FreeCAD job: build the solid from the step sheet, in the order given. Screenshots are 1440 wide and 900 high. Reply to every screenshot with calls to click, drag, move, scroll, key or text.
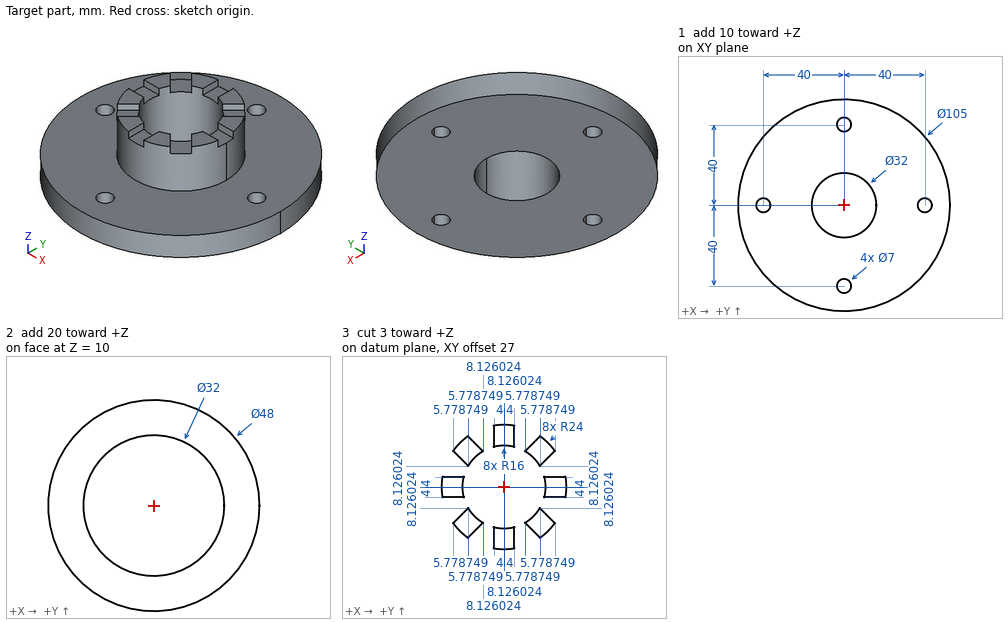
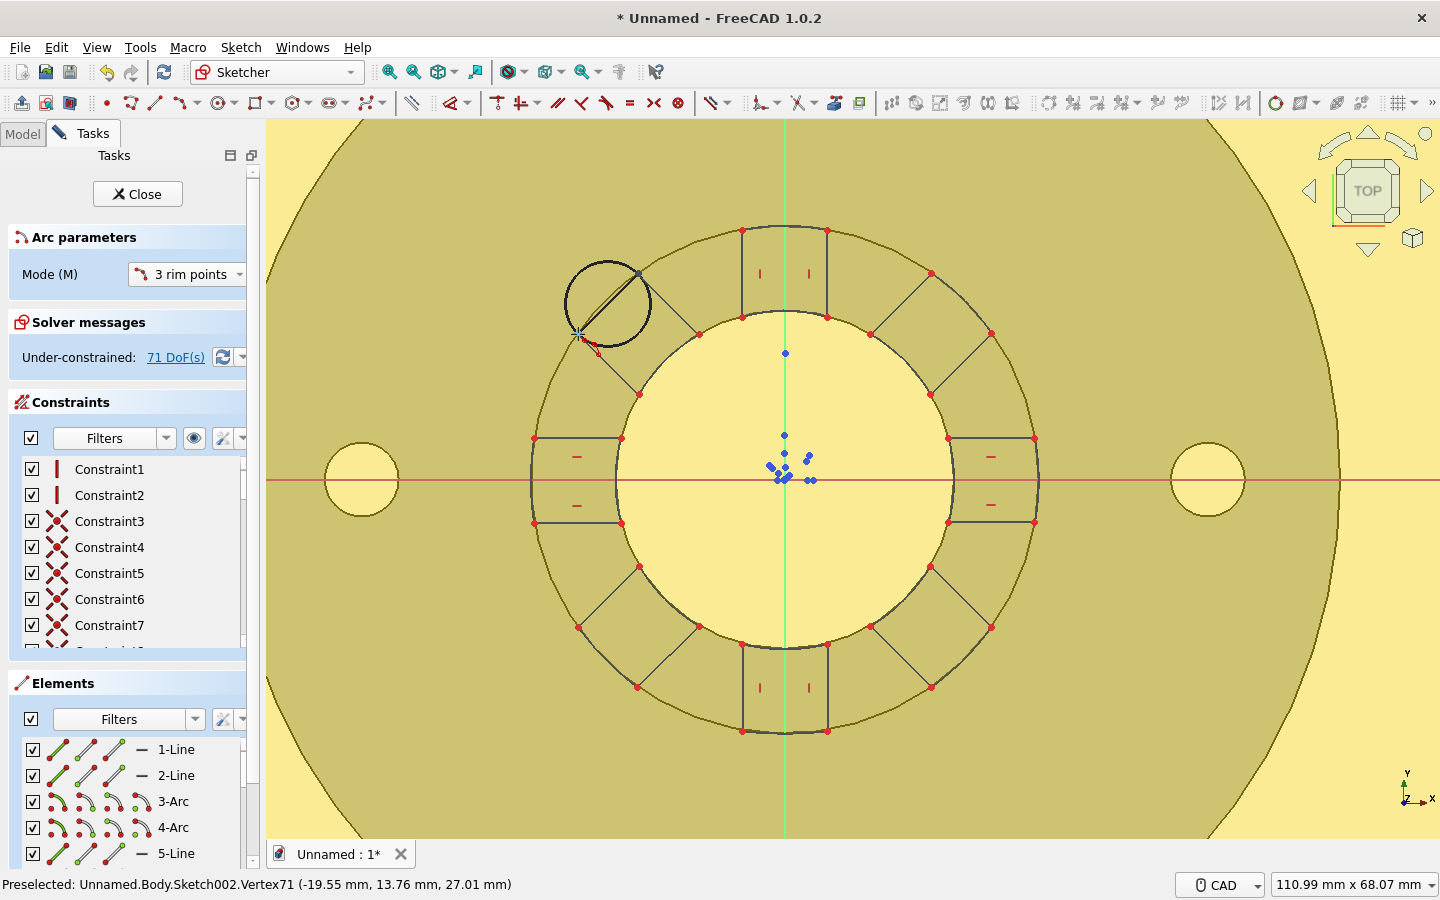
scroll(605, 300, up, 8)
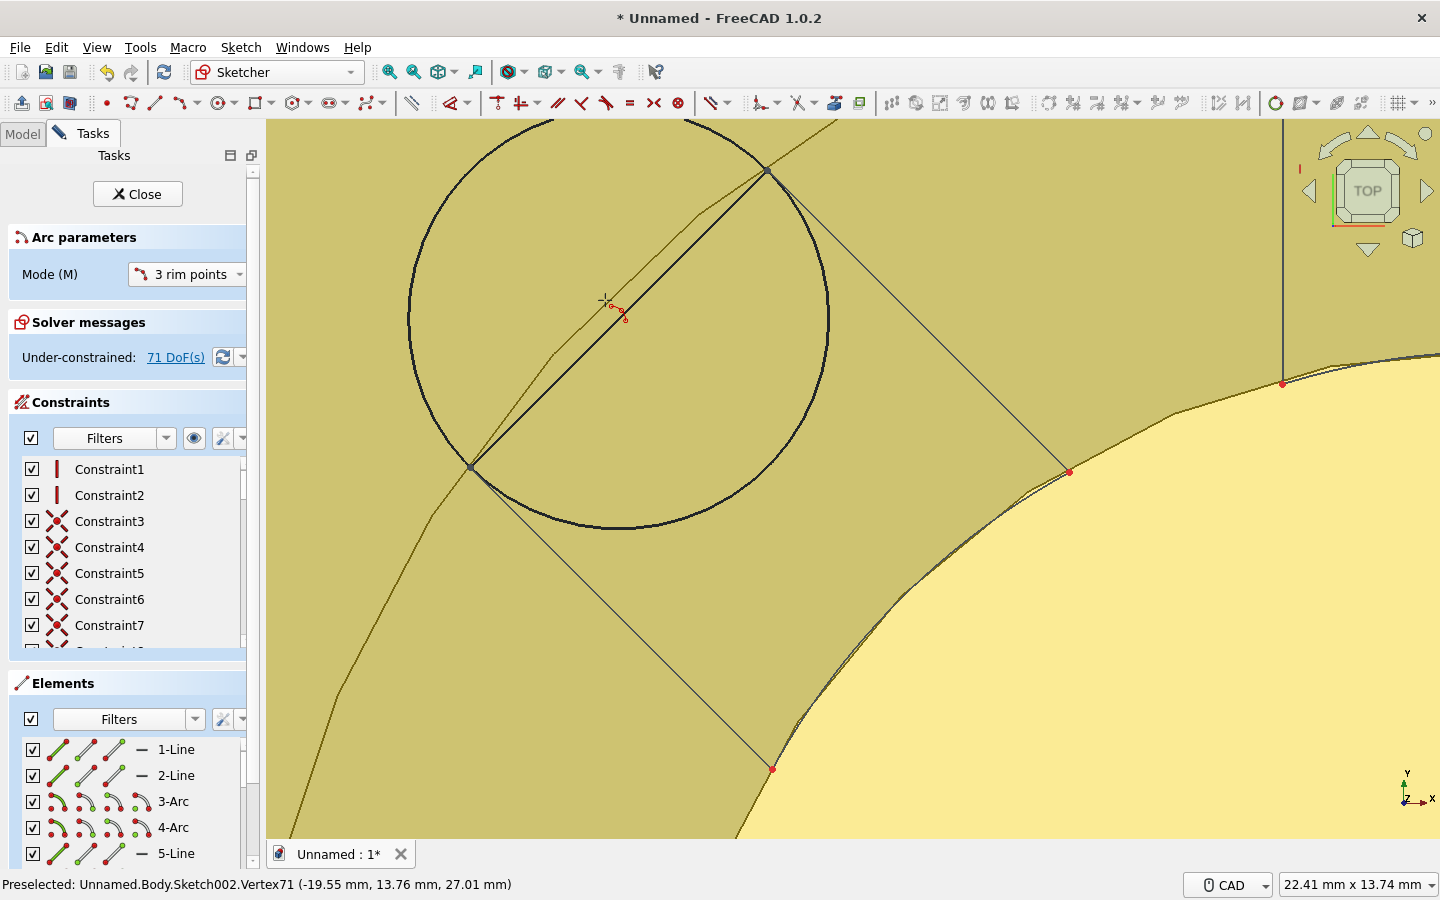
click(605, 299)
key(Escape)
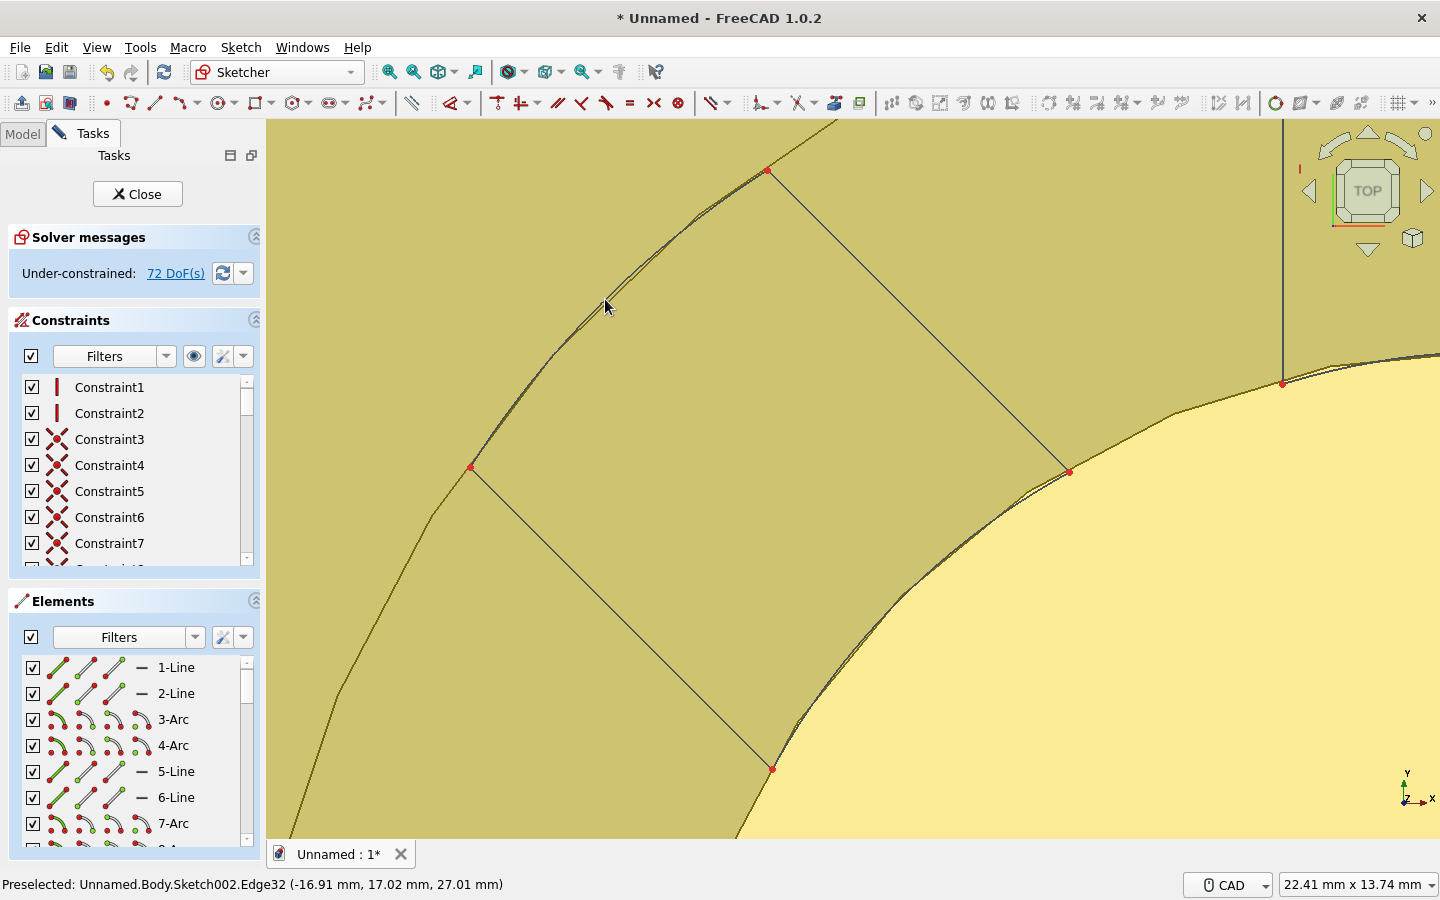
scroll(605, 300, down, 8)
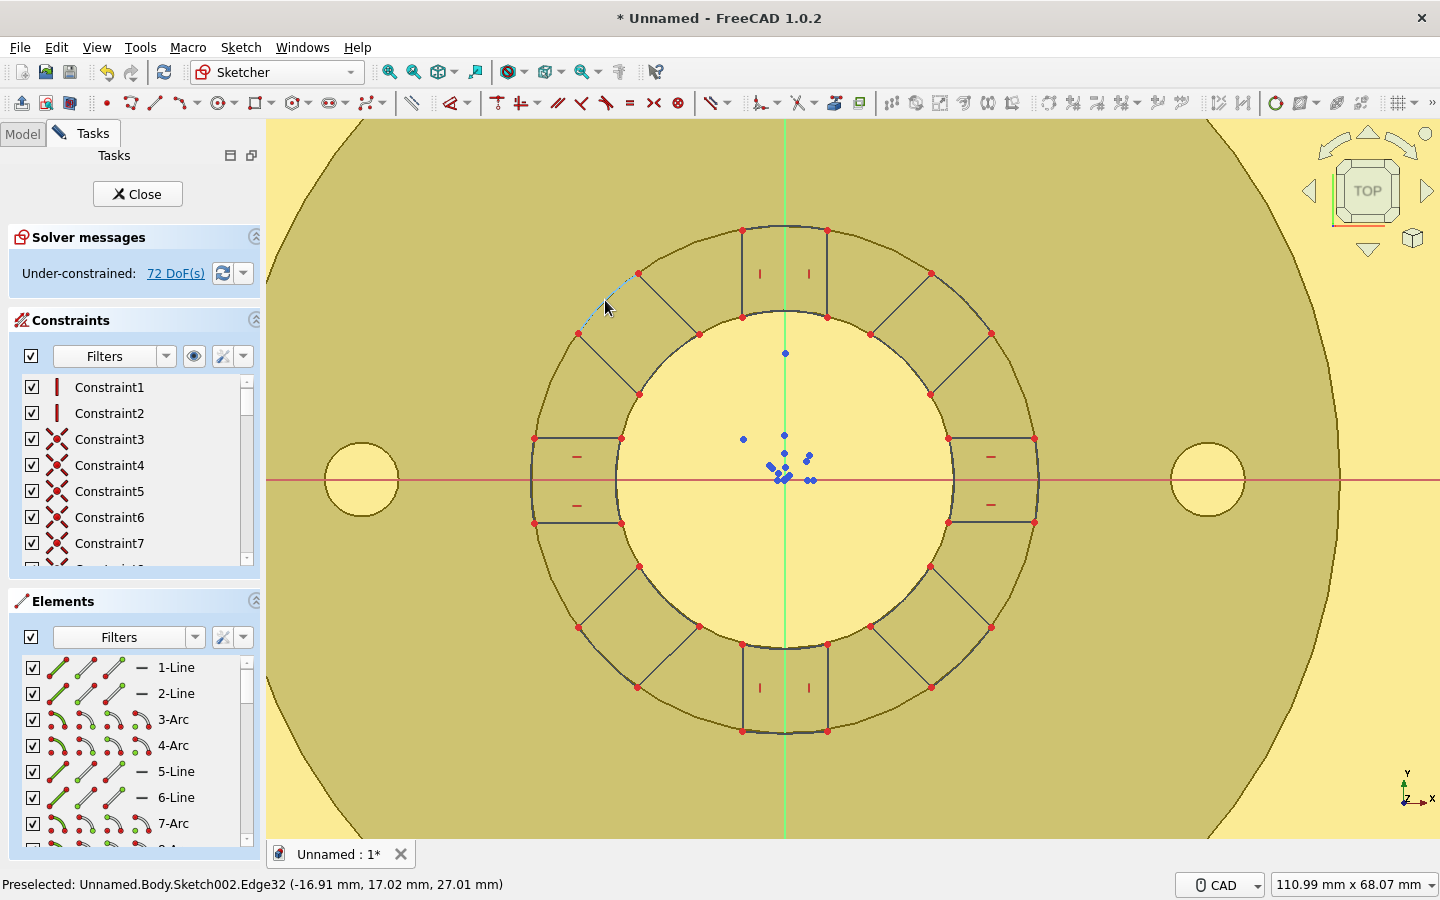
click(802, 312)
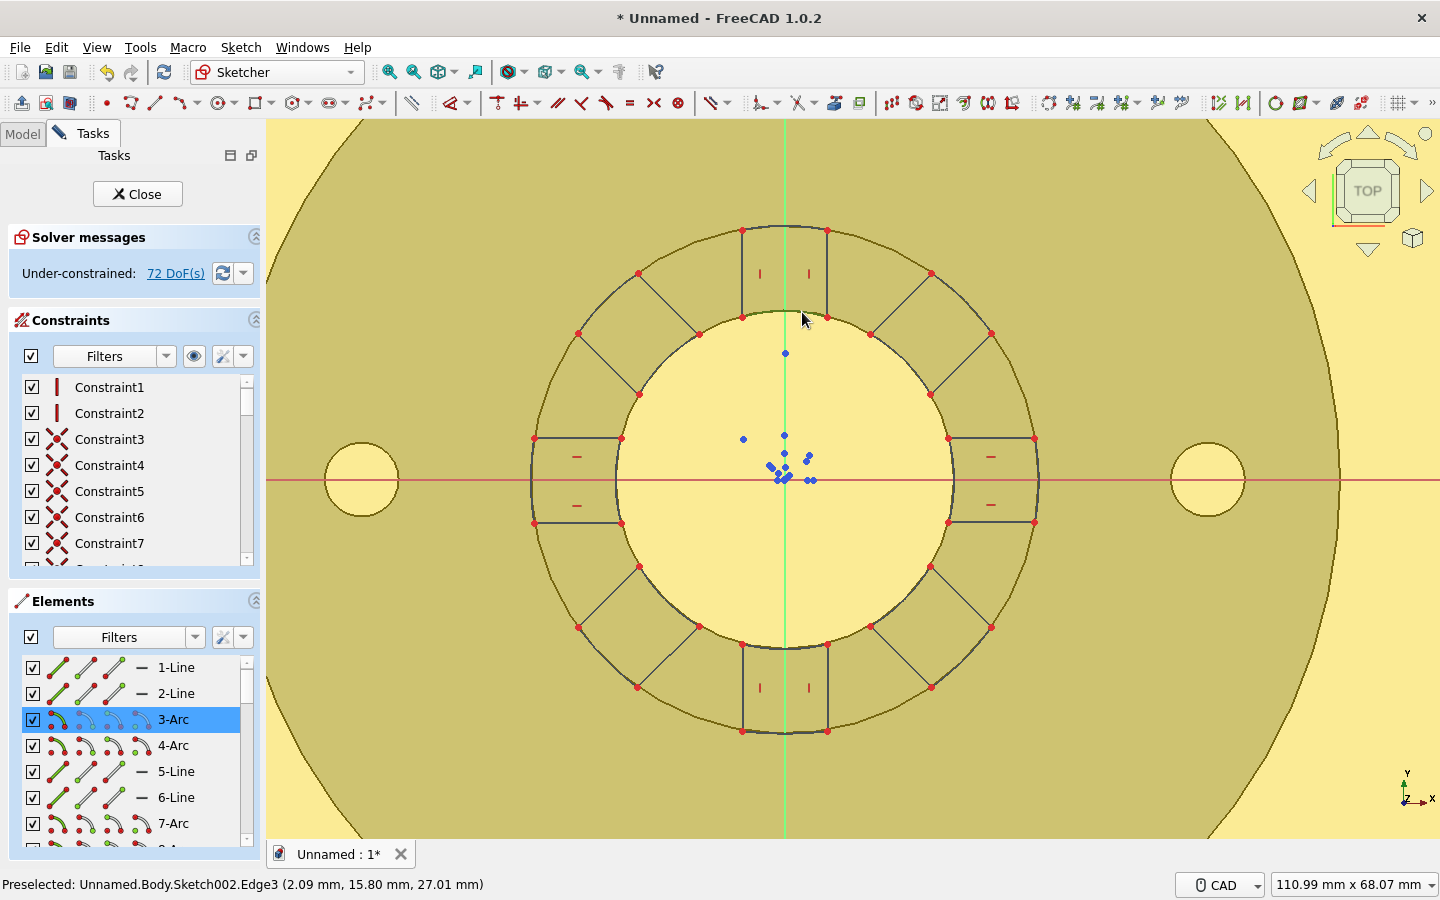
click(802, 227)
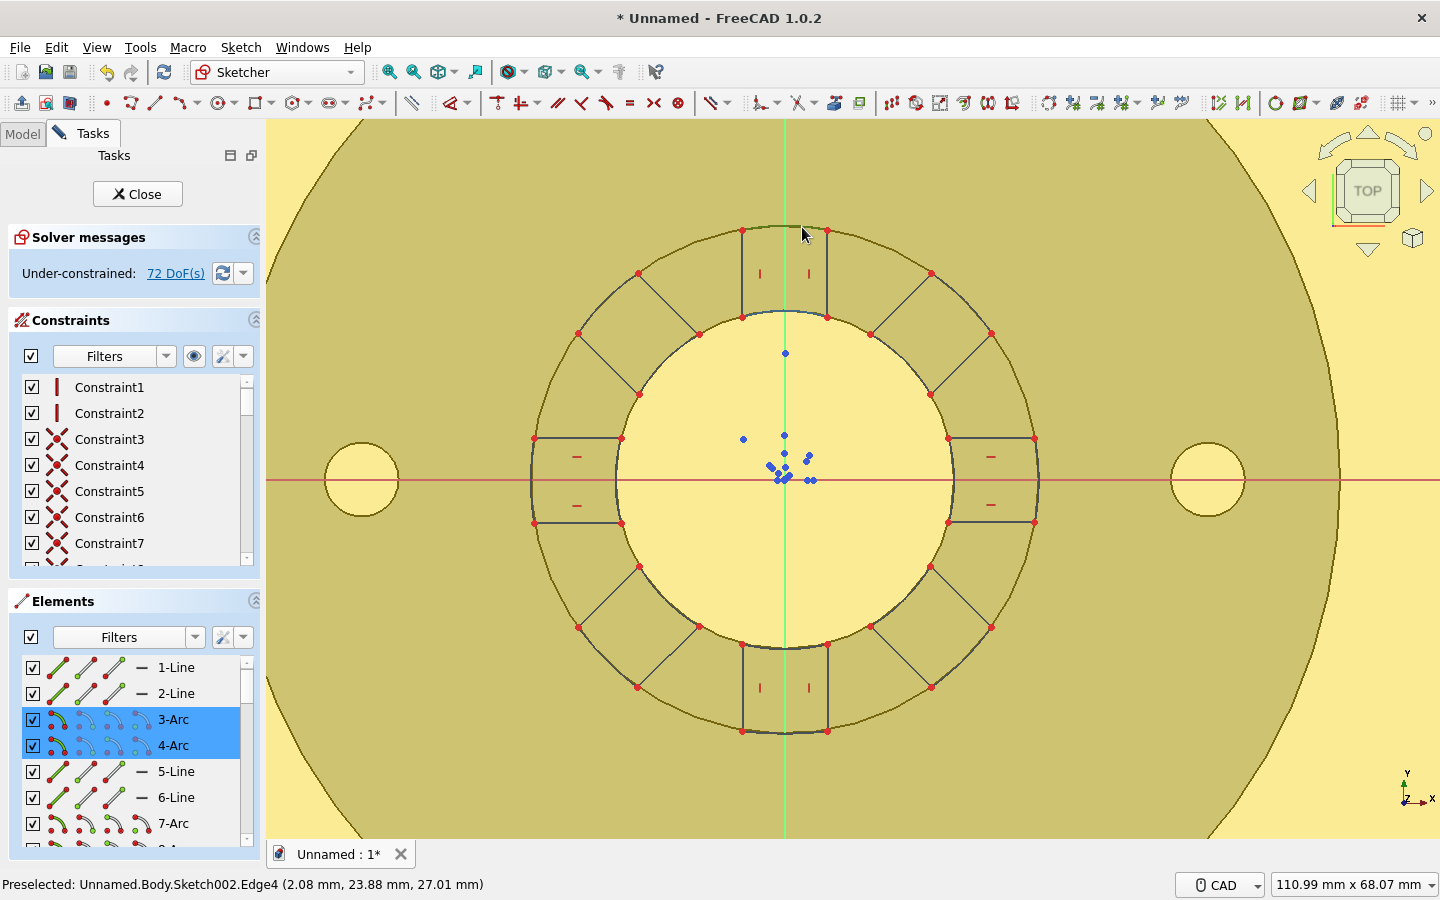
click(498, 104)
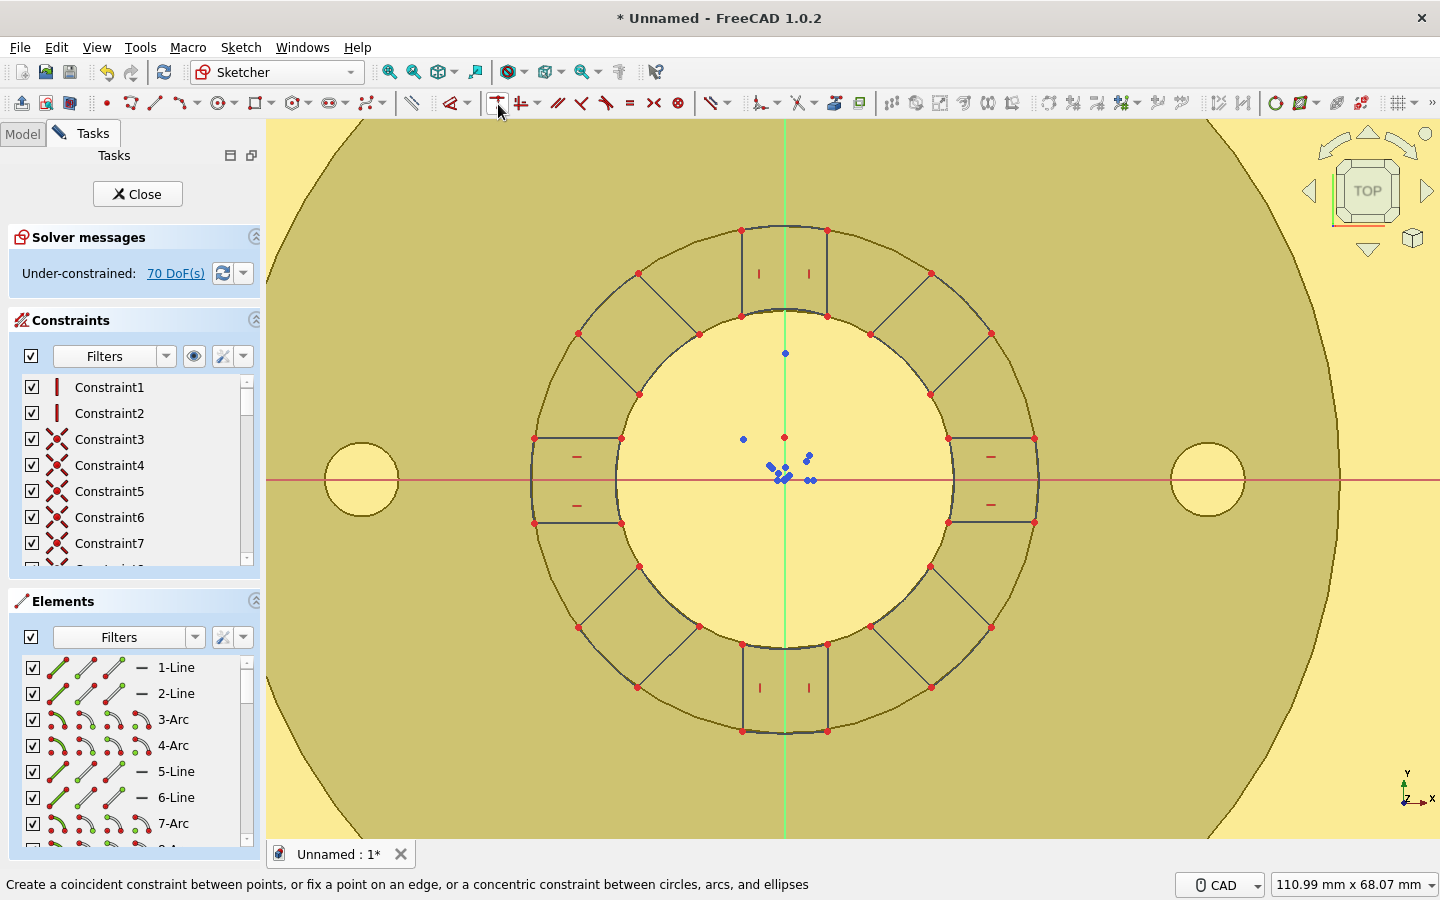
click(802, 310)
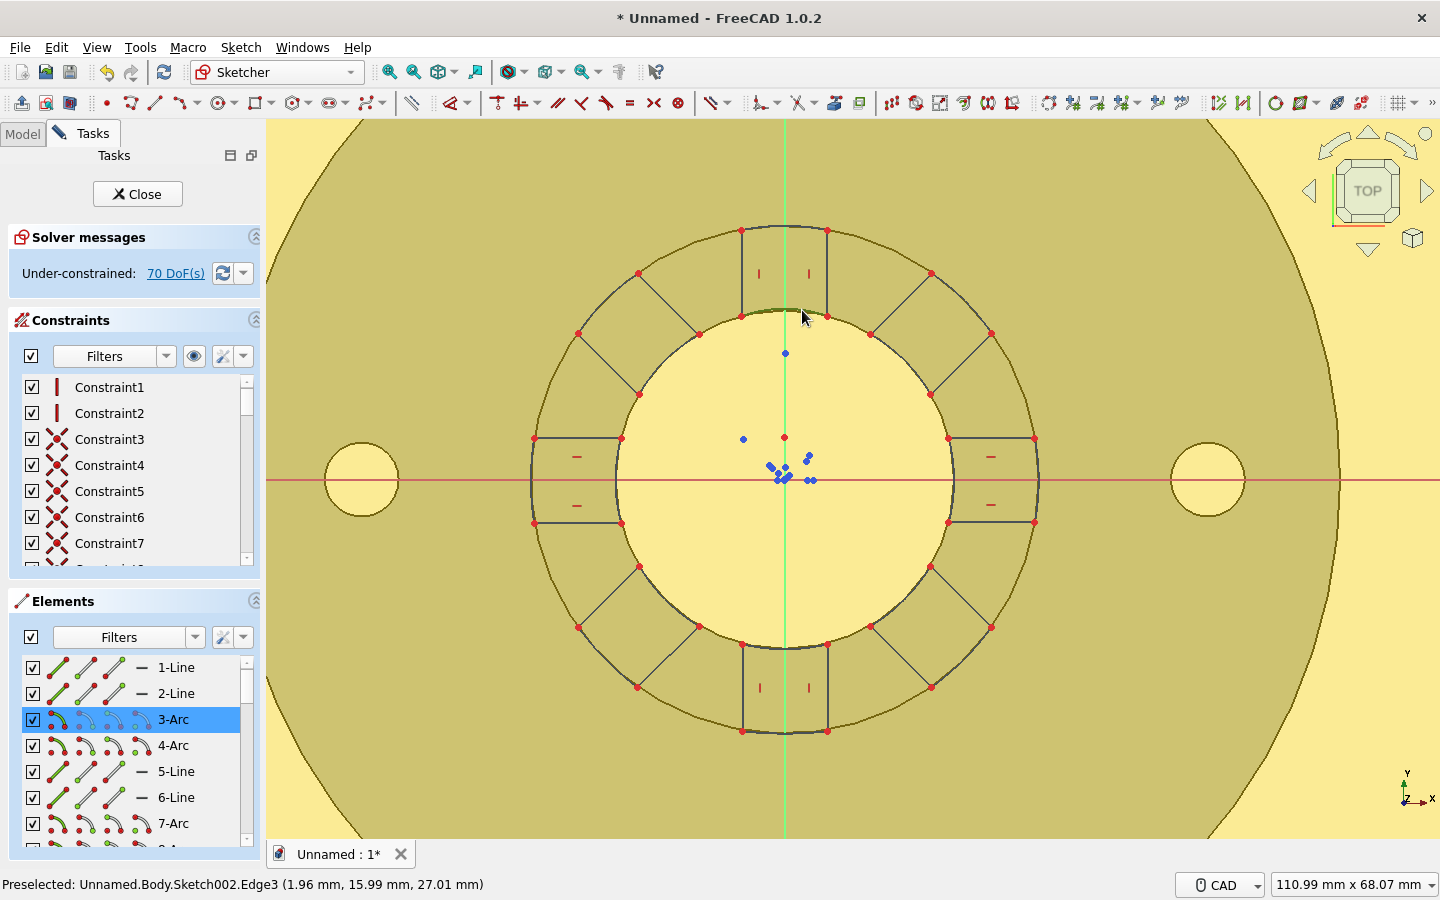
click(916, 373)